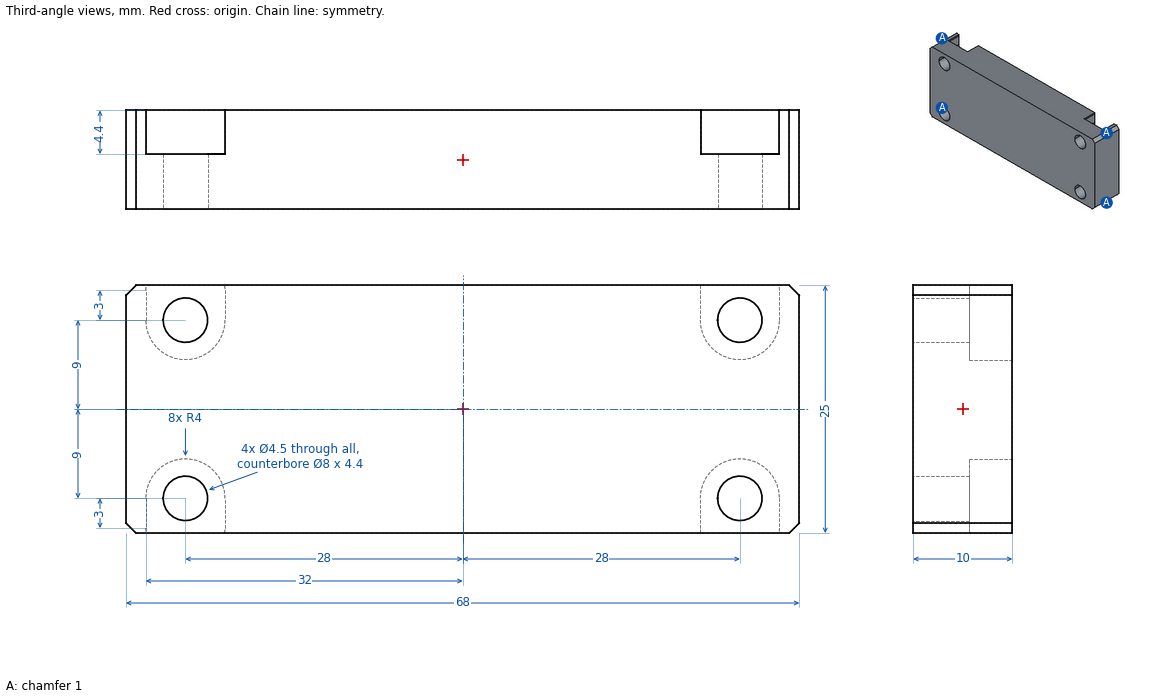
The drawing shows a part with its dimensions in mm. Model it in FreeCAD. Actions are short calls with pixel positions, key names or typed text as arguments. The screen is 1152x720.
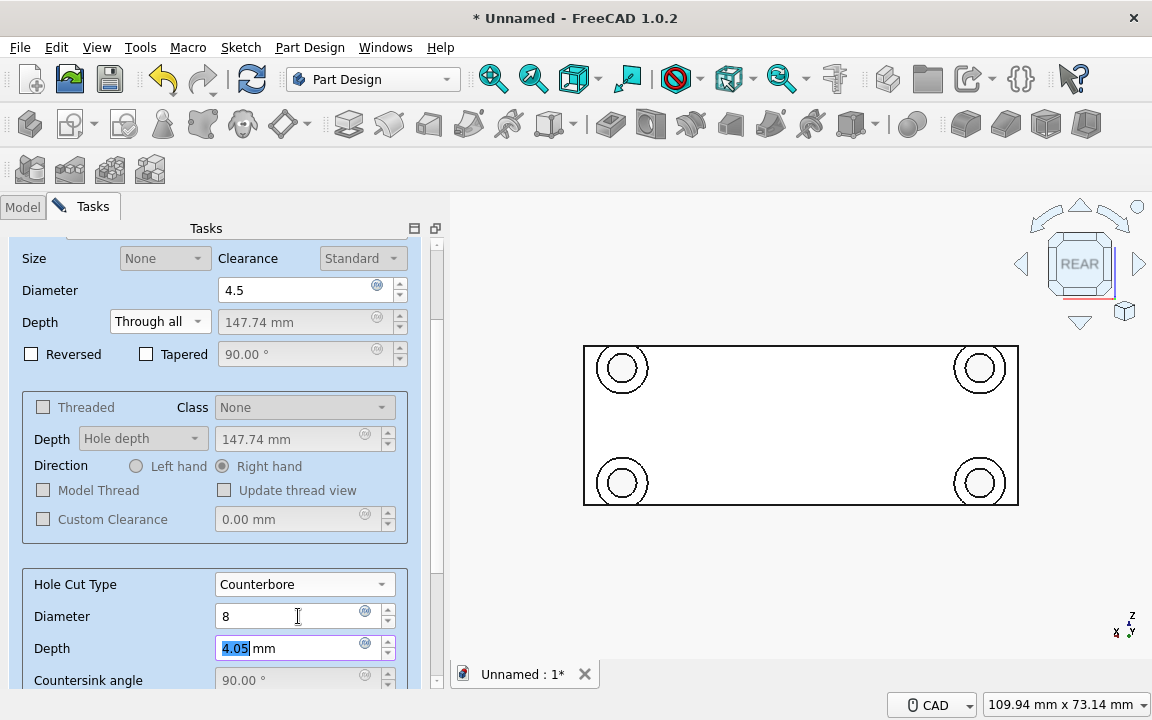
text(4.4)
key(Tab)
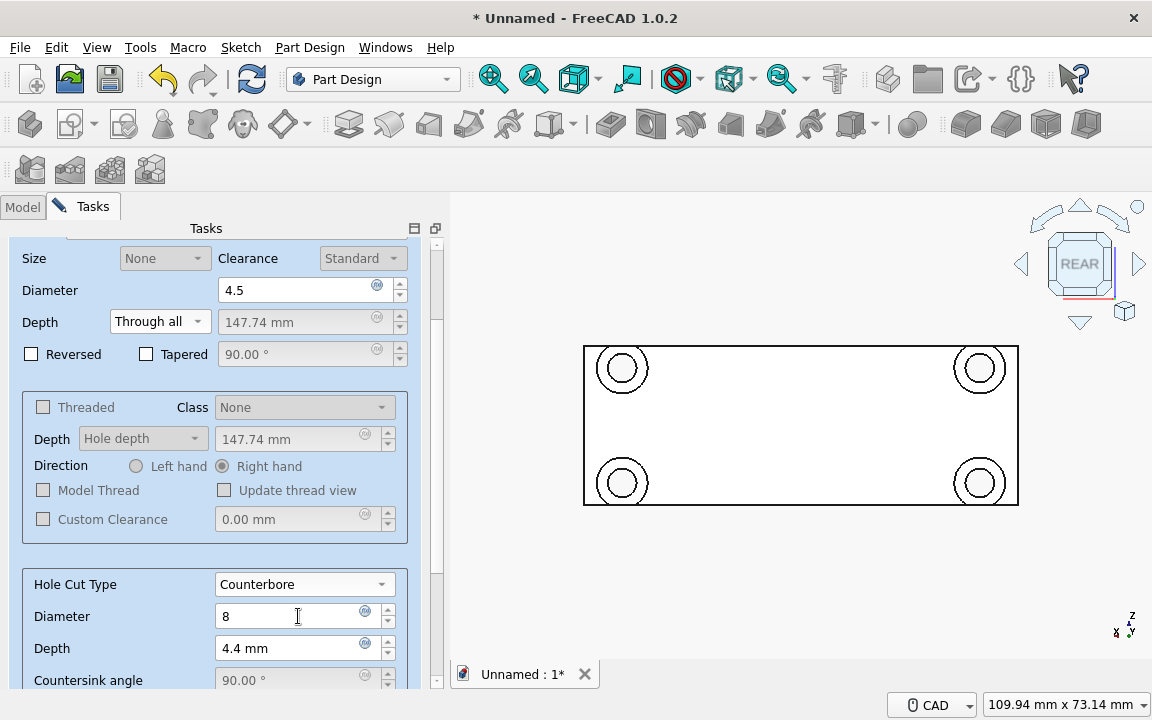
scroll(437, 463, up, 3)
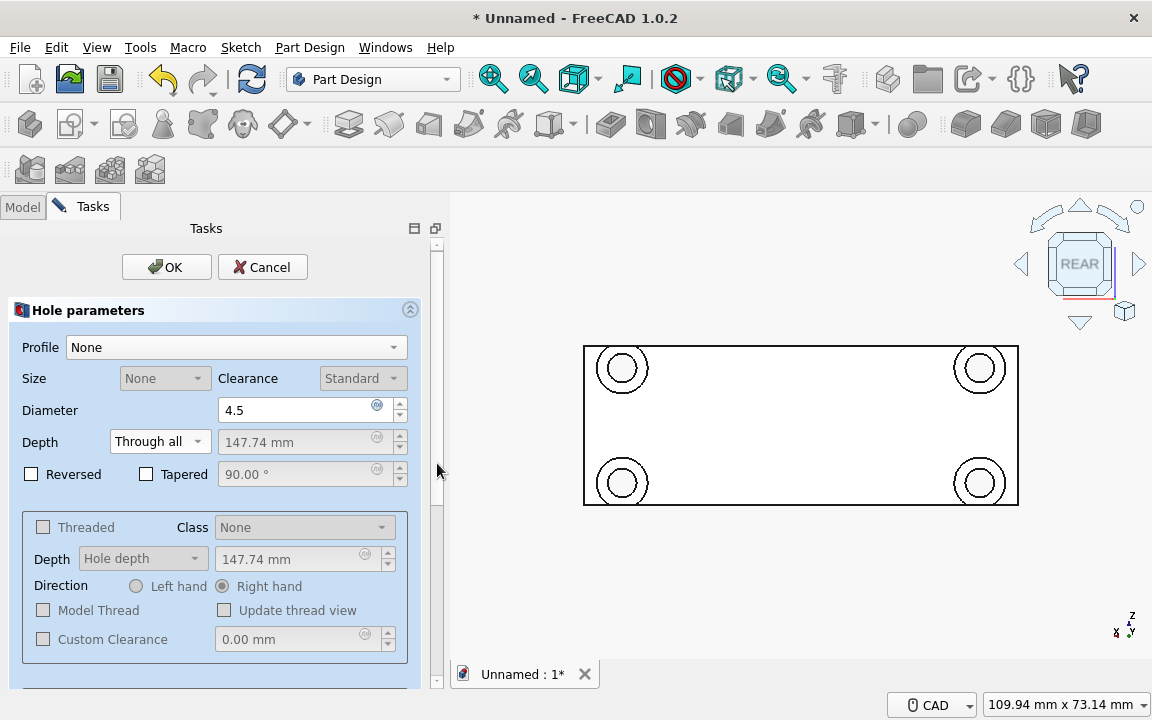
click(167, 267)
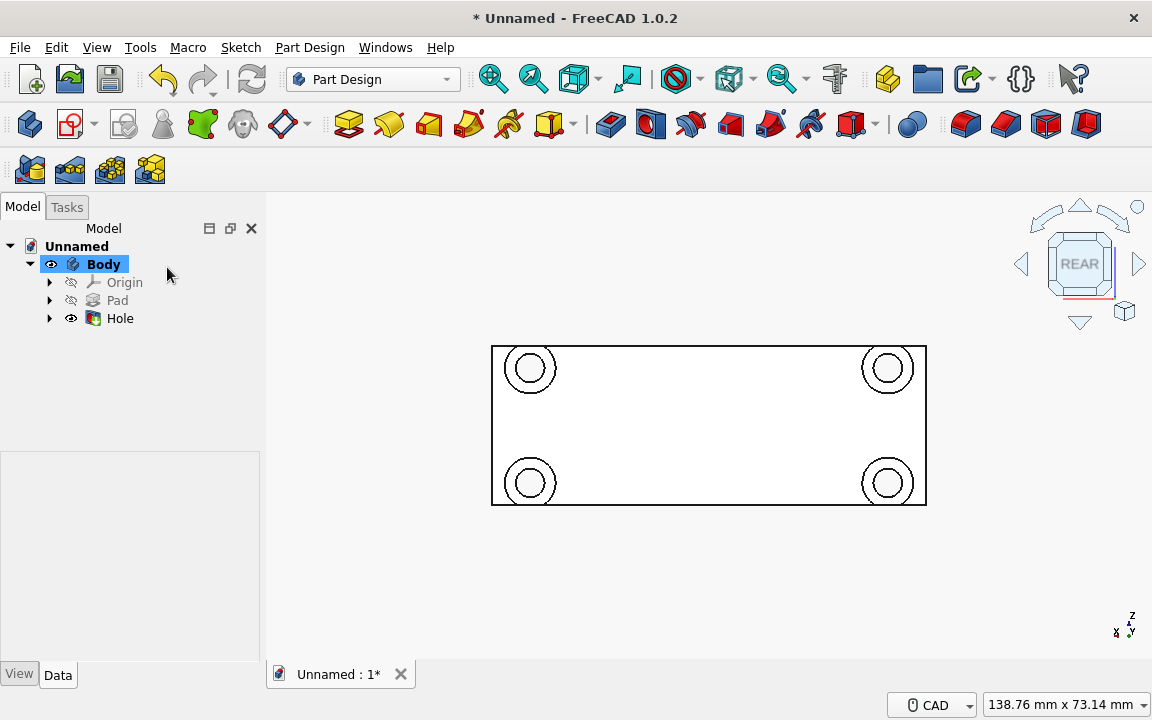
click(647, 424)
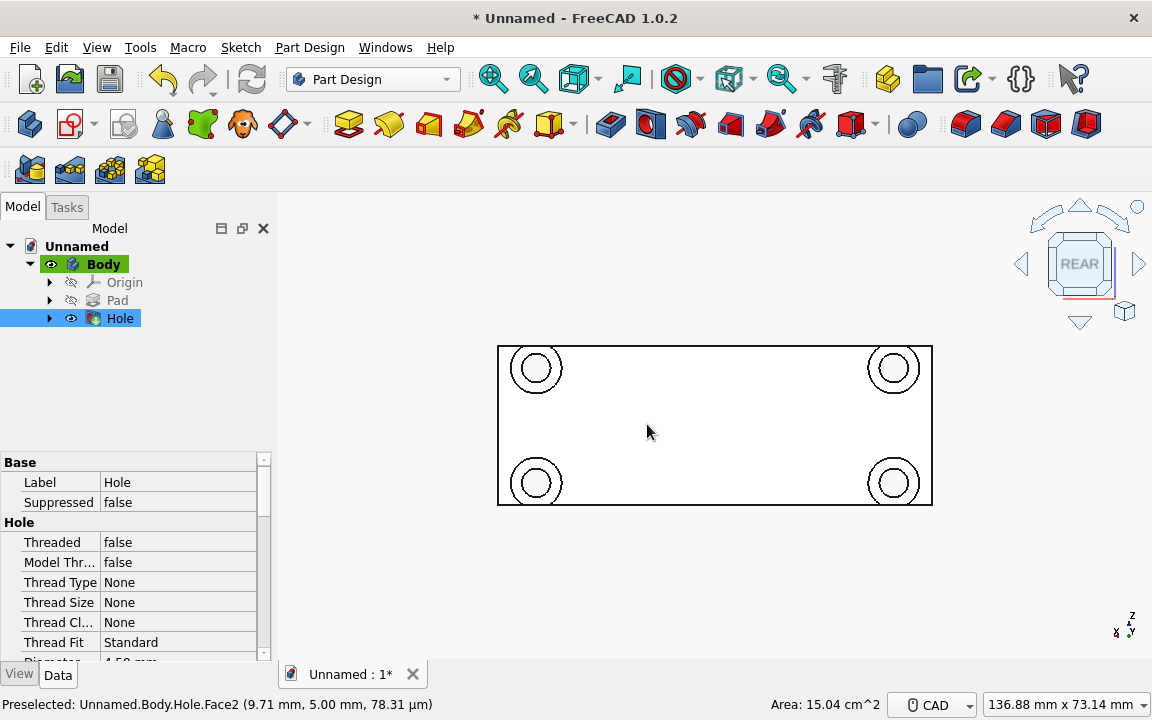
click(70, 124)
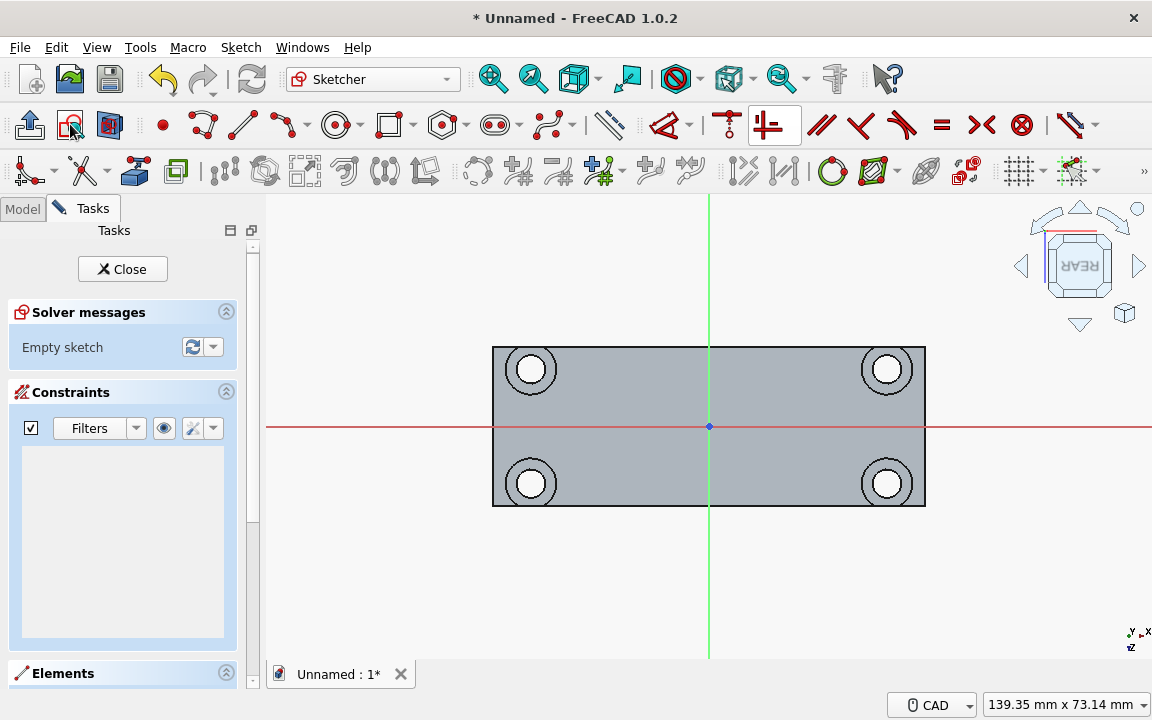
click(496, 126)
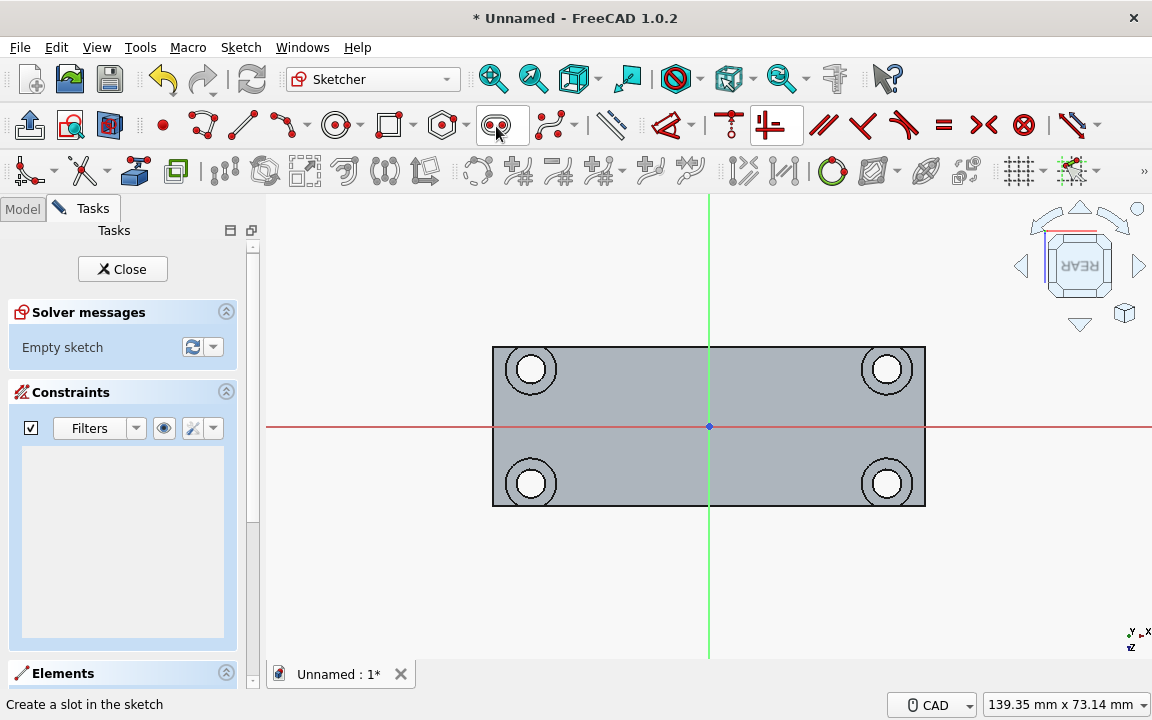
click(531, 369)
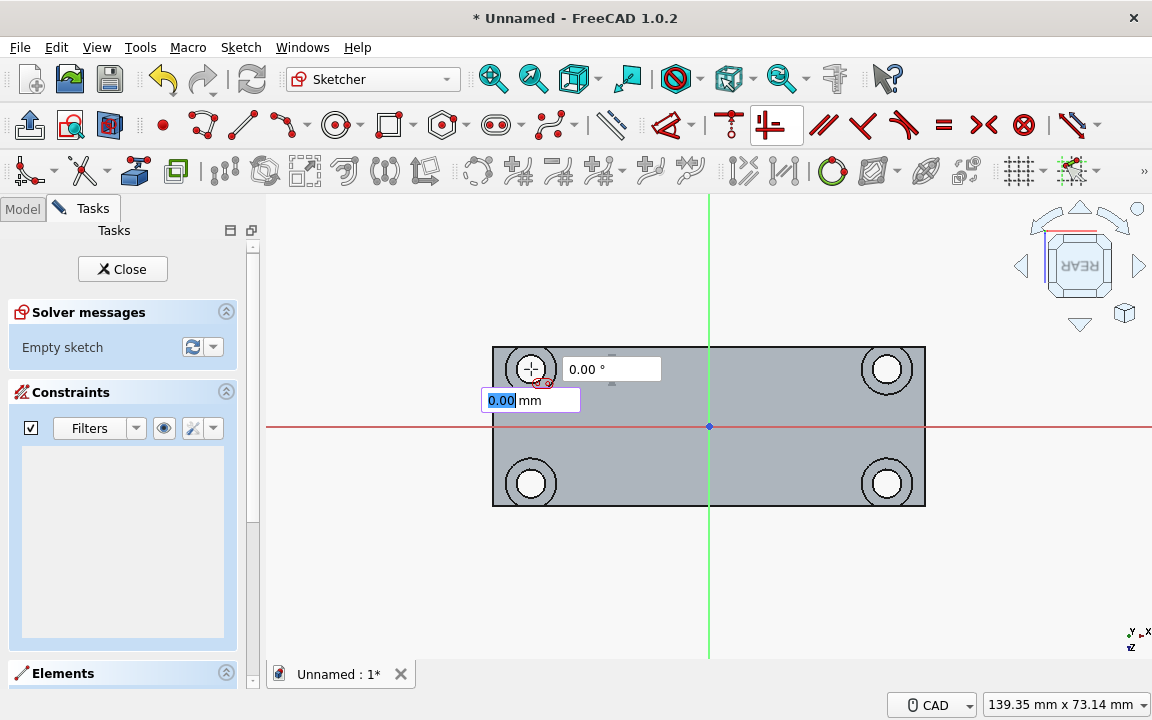
click(531, 350)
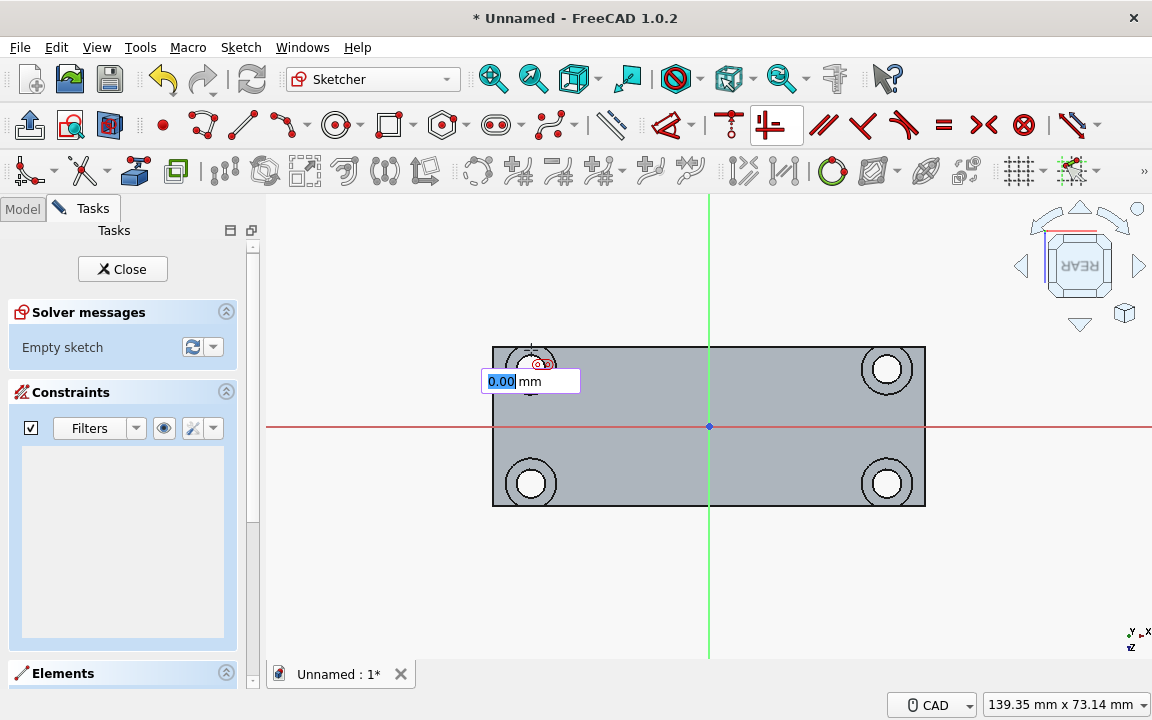
click(506, 360)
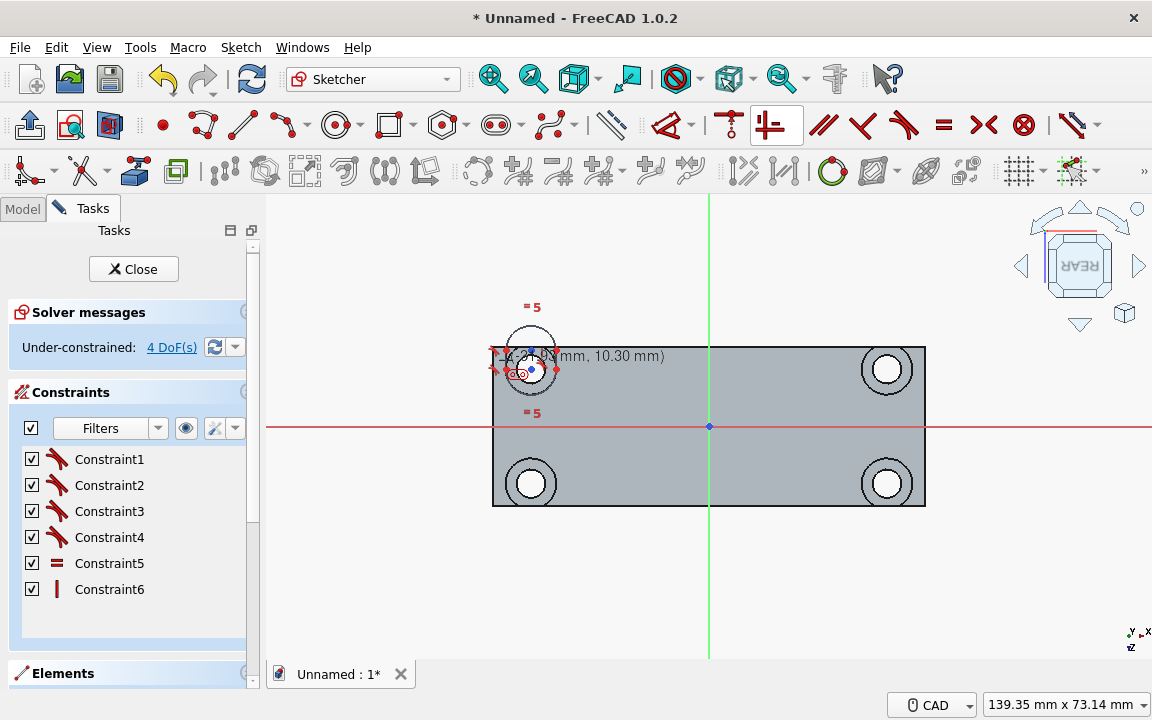
click(531, 503)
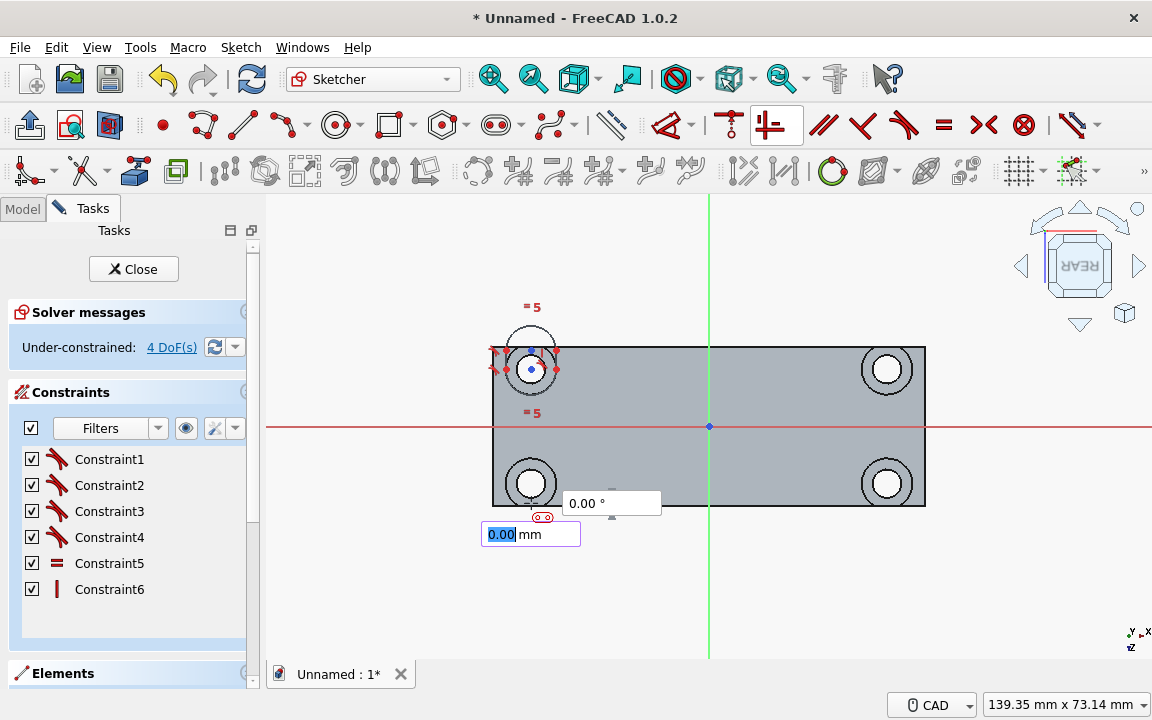
click(531, 484)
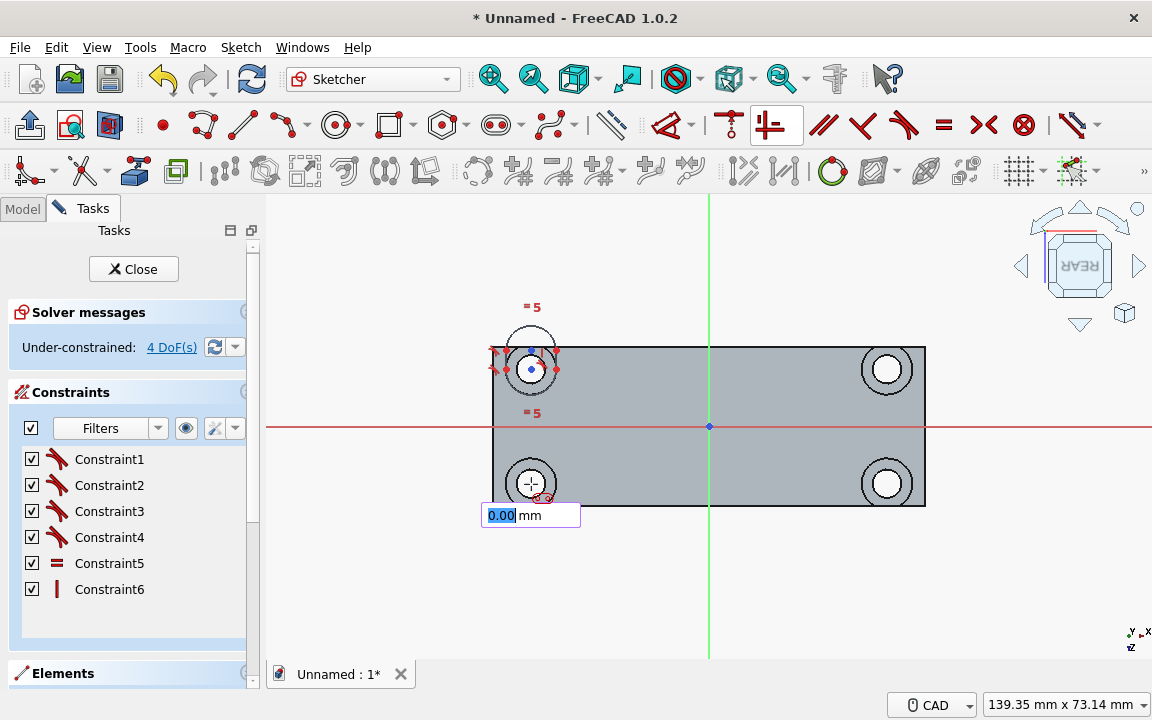
click(506, 493)